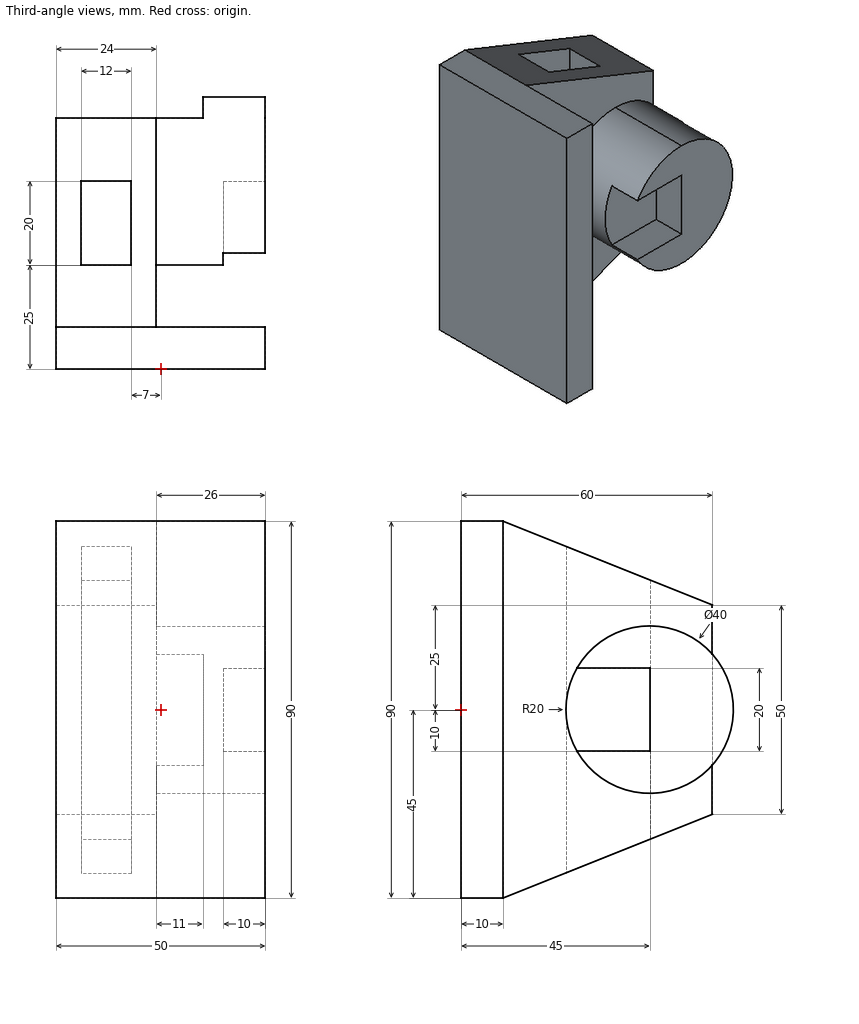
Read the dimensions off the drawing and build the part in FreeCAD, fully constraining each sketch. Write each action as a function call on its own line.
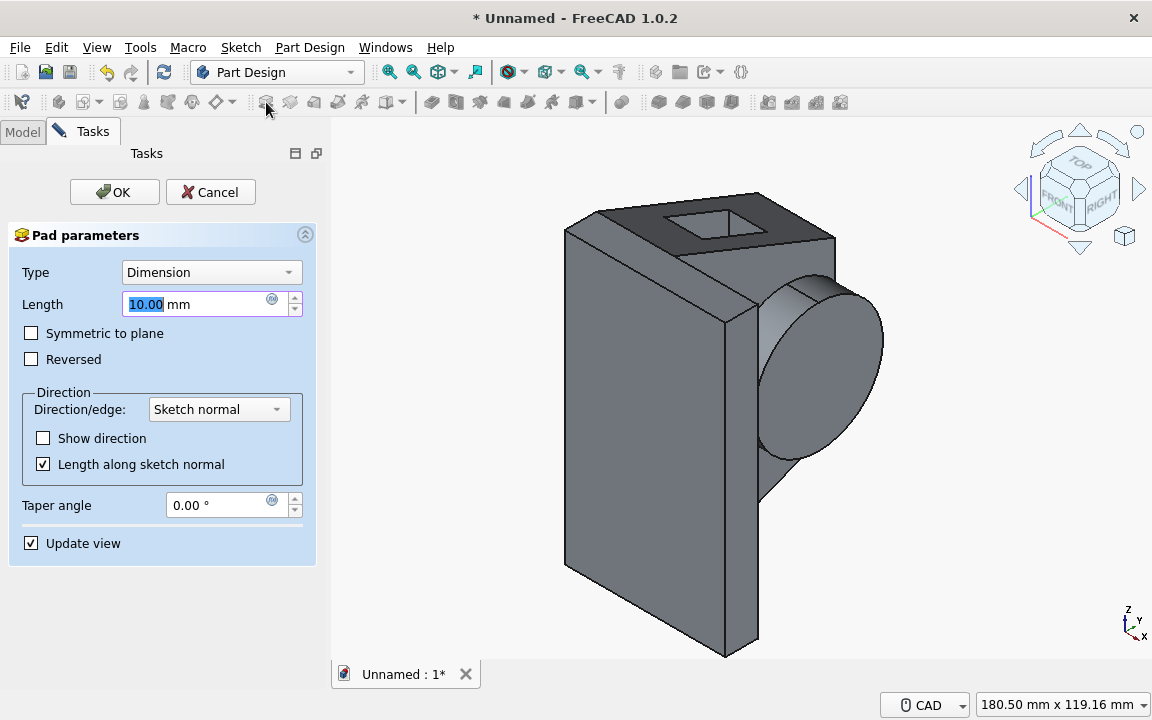
text(26)
key(Tab)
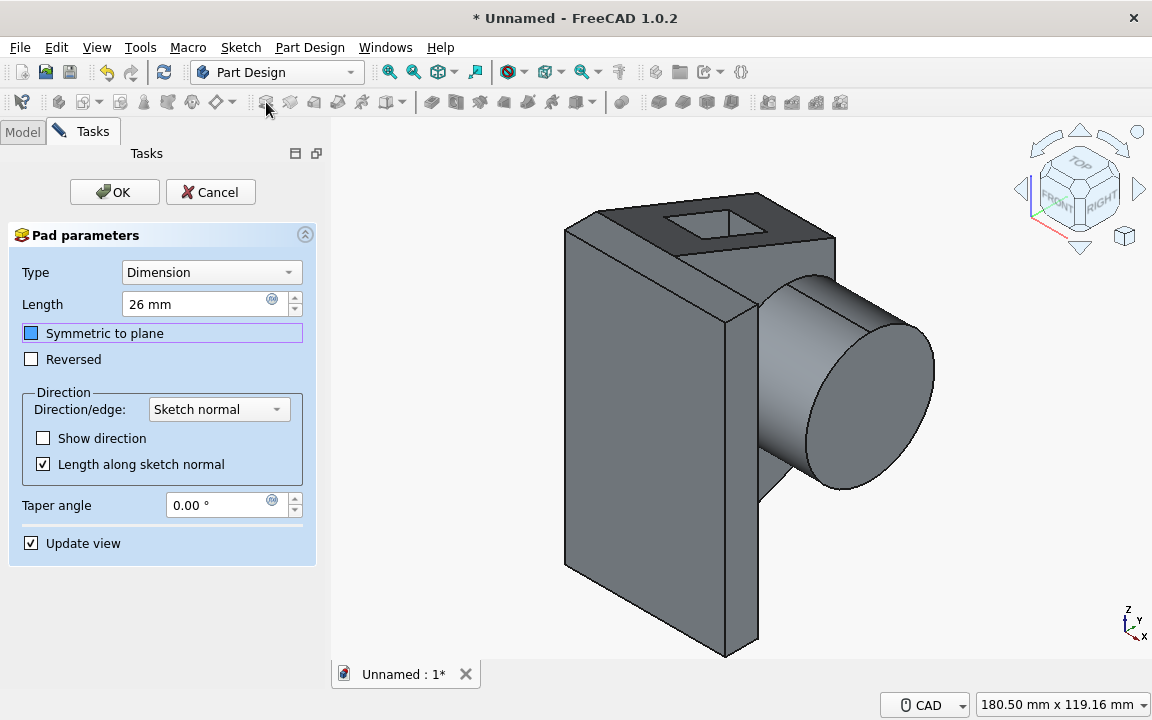
click(115, 192)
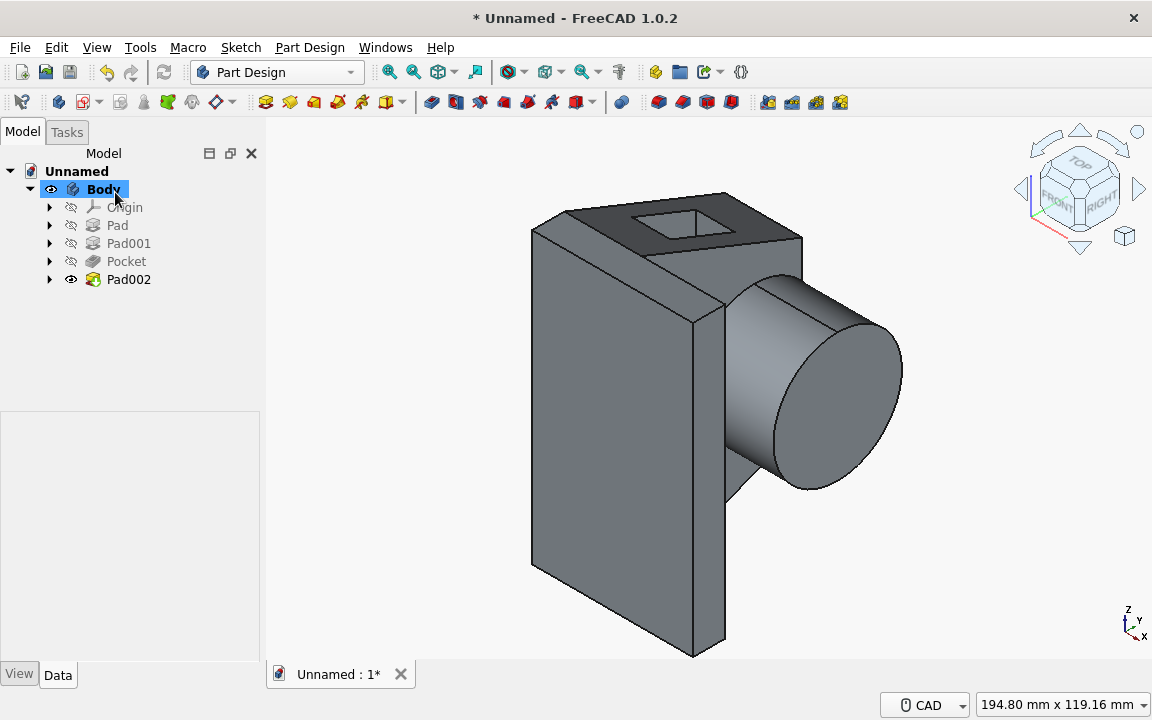
click(390, 72)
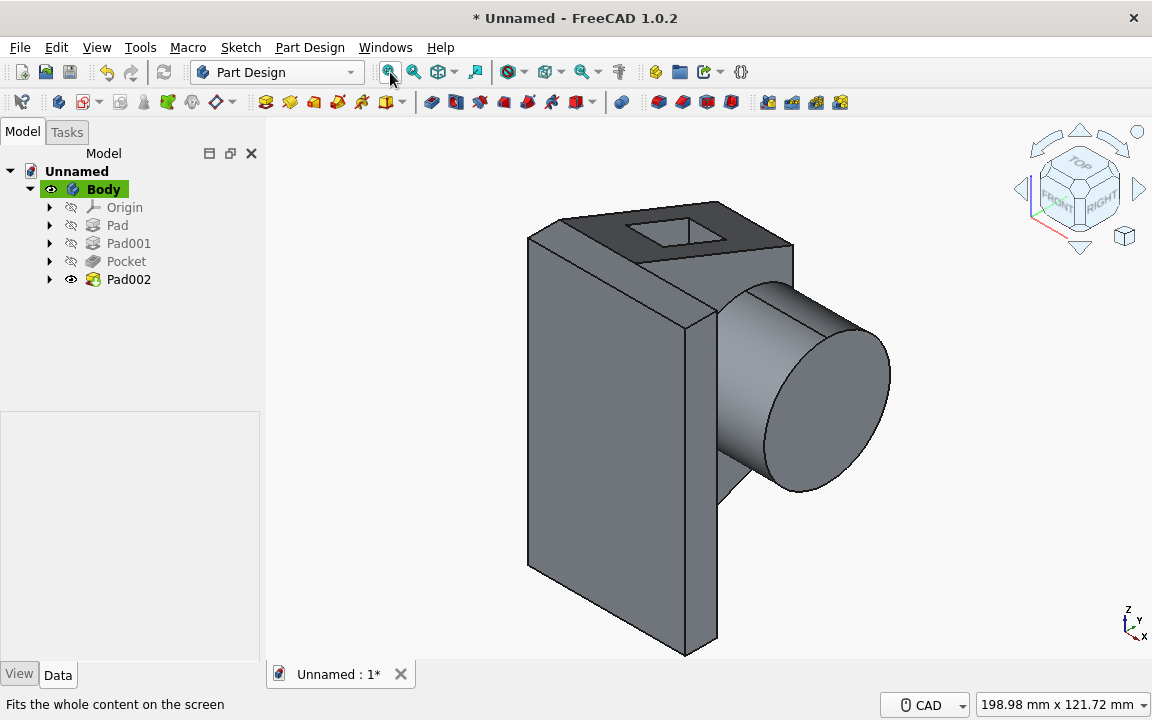
click(50, 207)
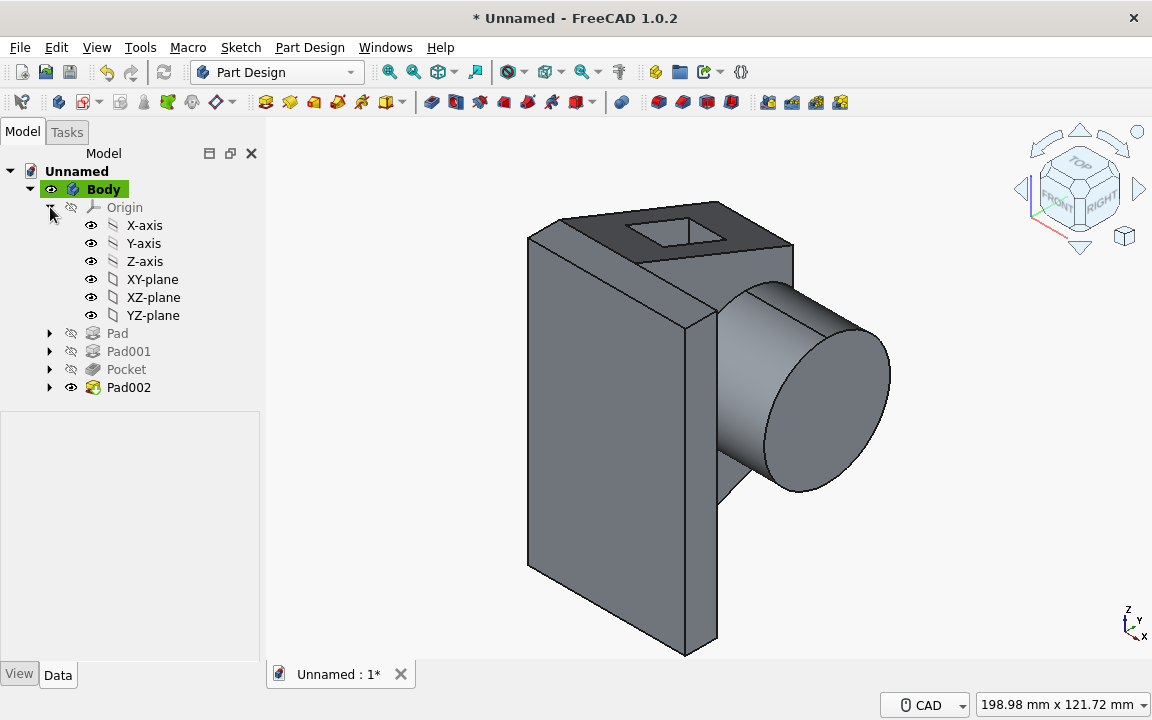
click(136, 315)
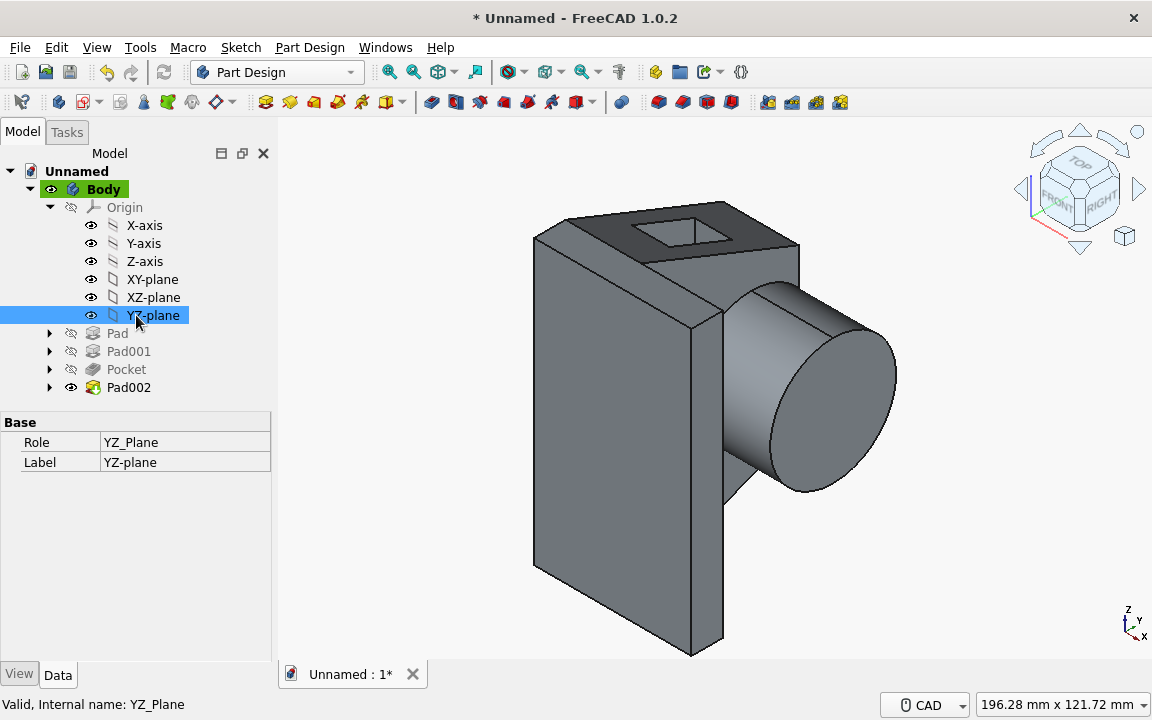
click(216, 102)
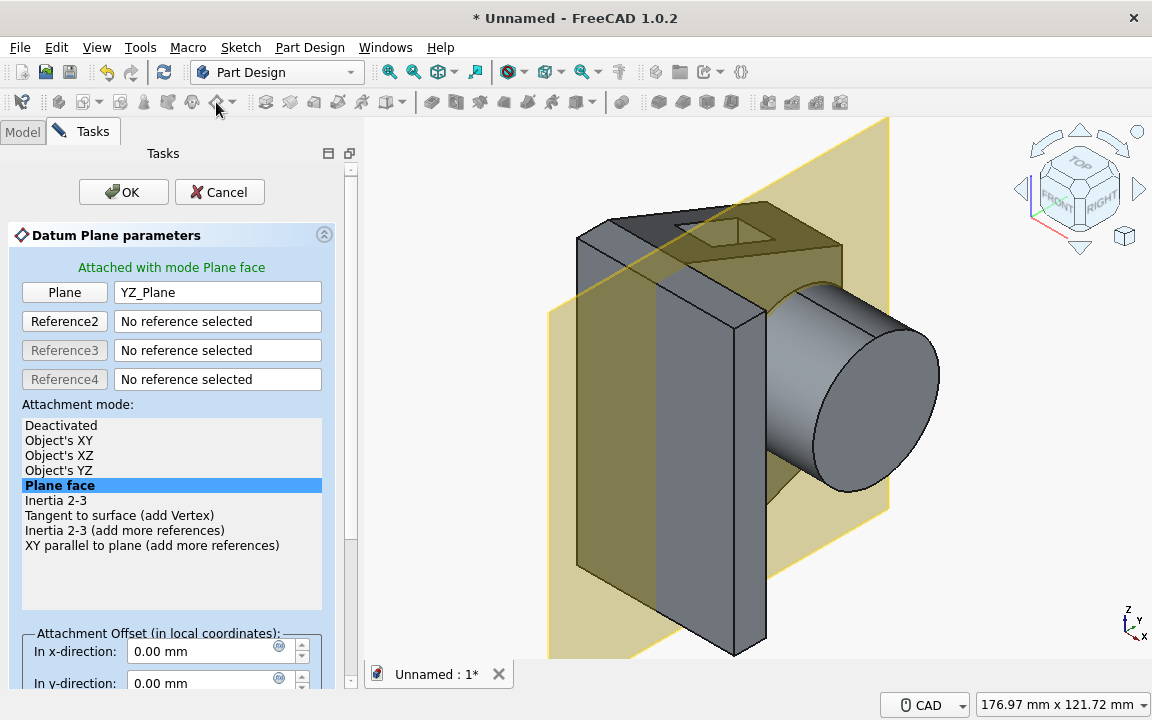
scroll(351, 426, down, 2)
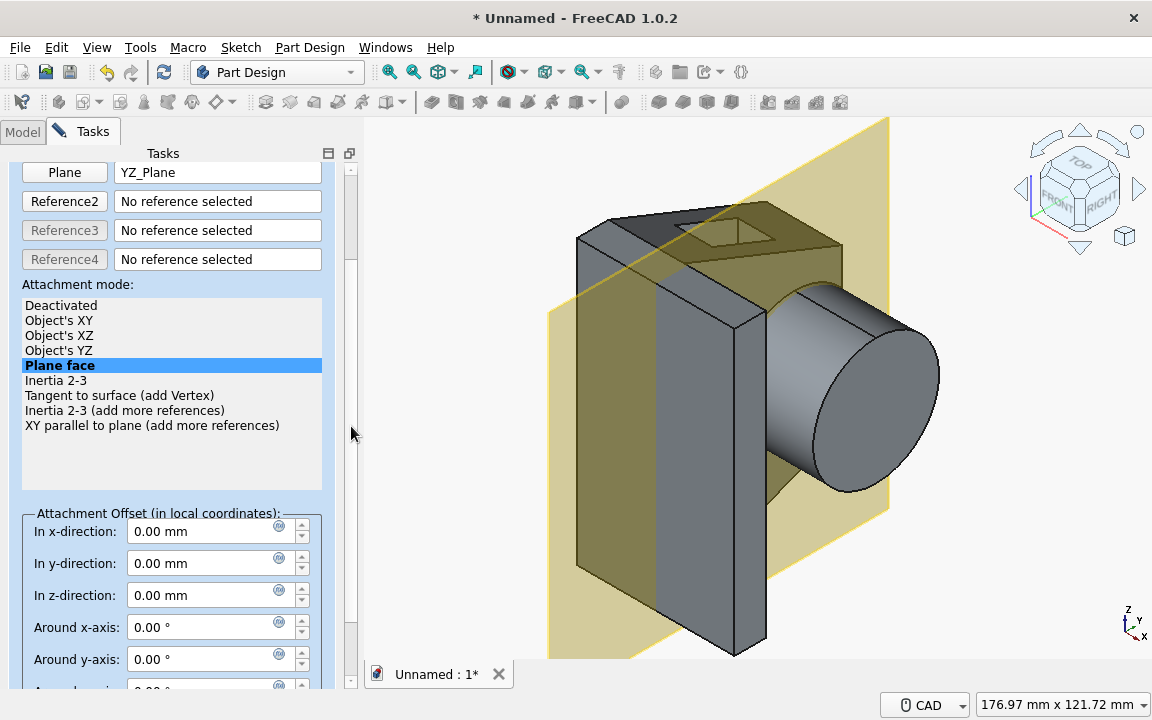
triple_click(210, 595)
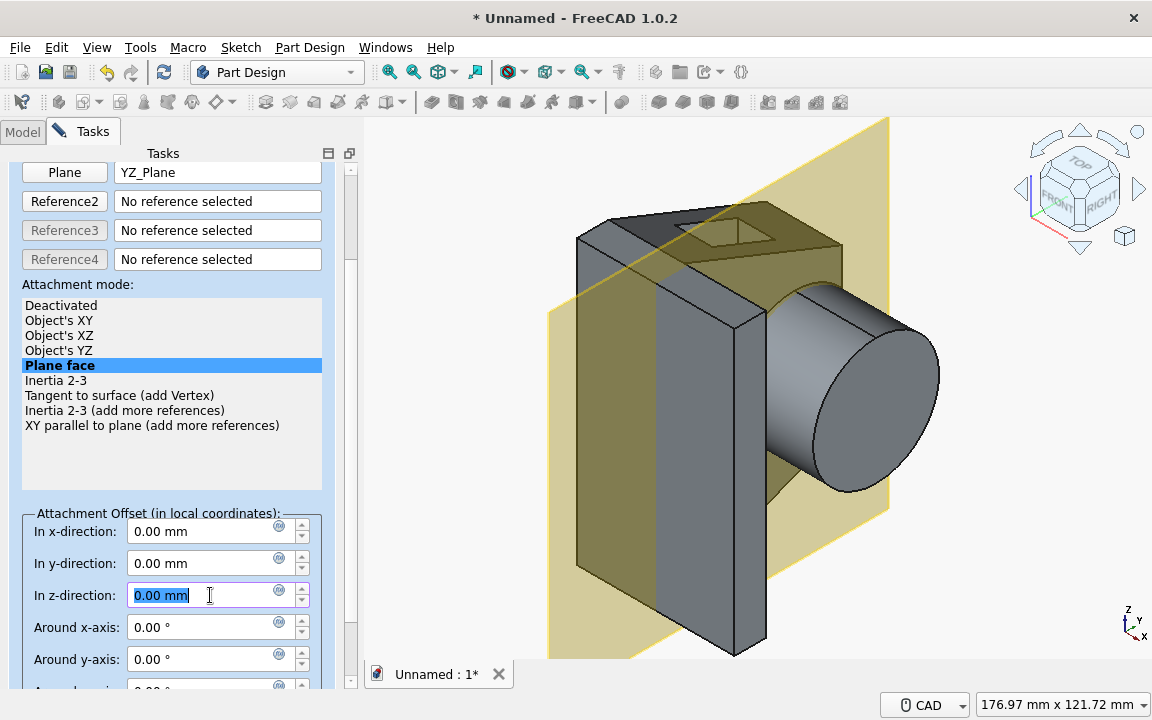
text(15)
key(Tab)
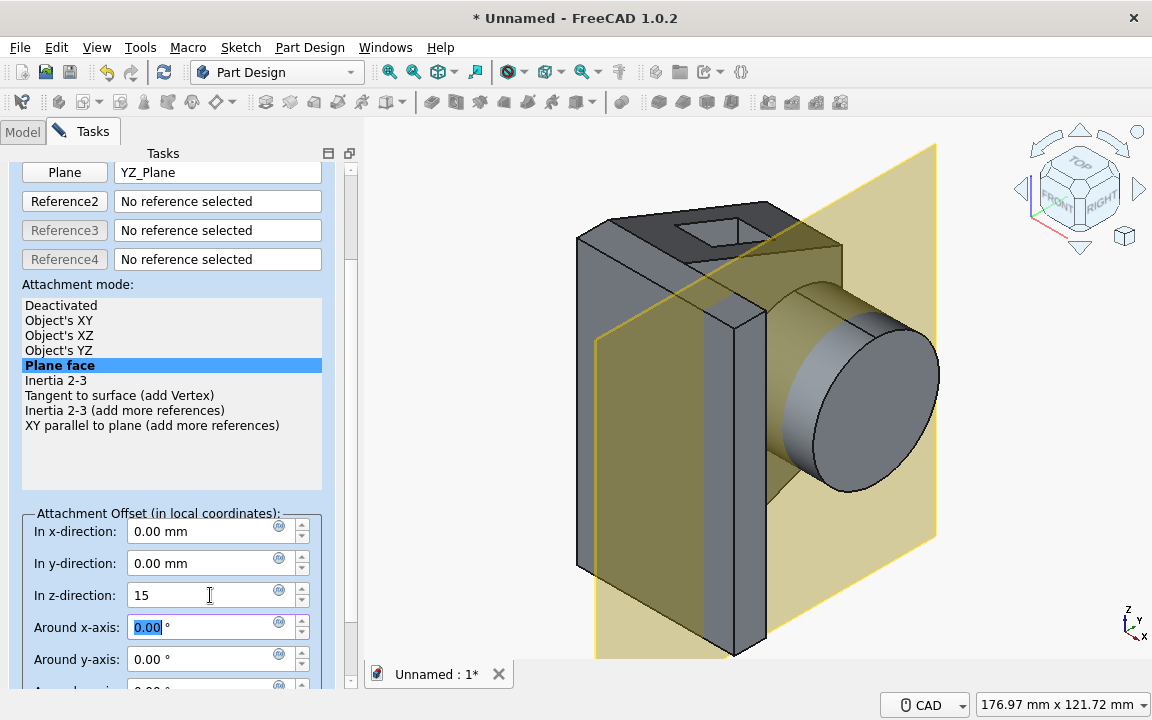
scroll(351, 426, up, 3)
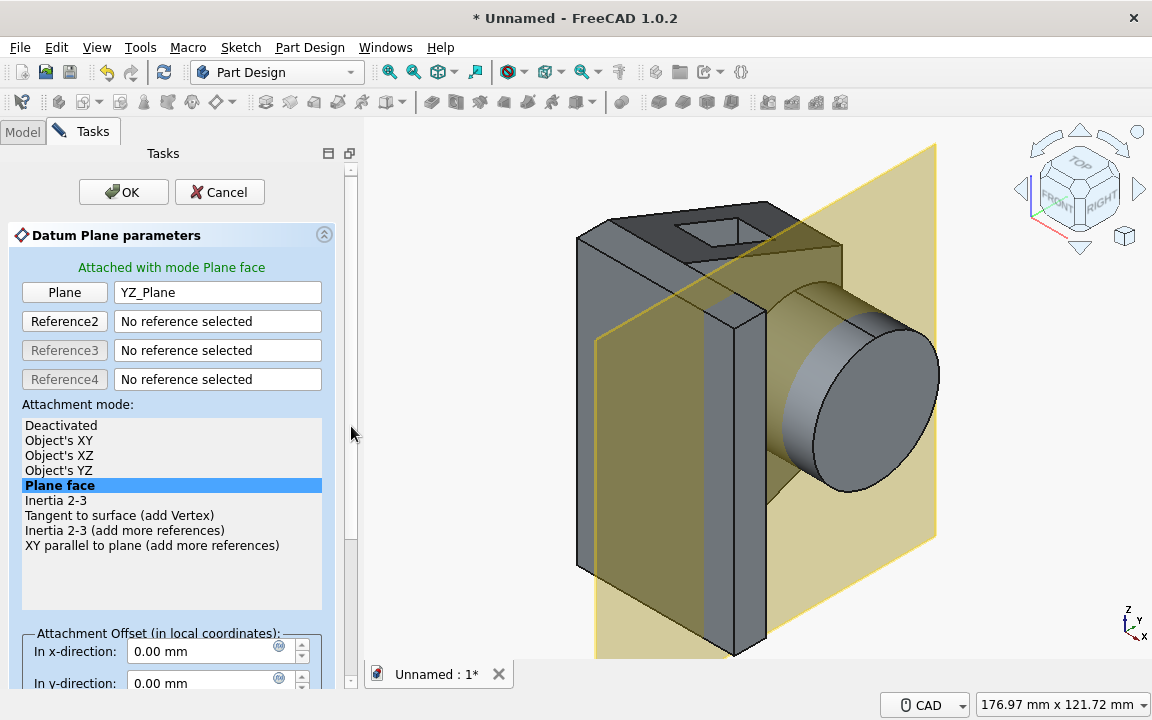
click(124, 192)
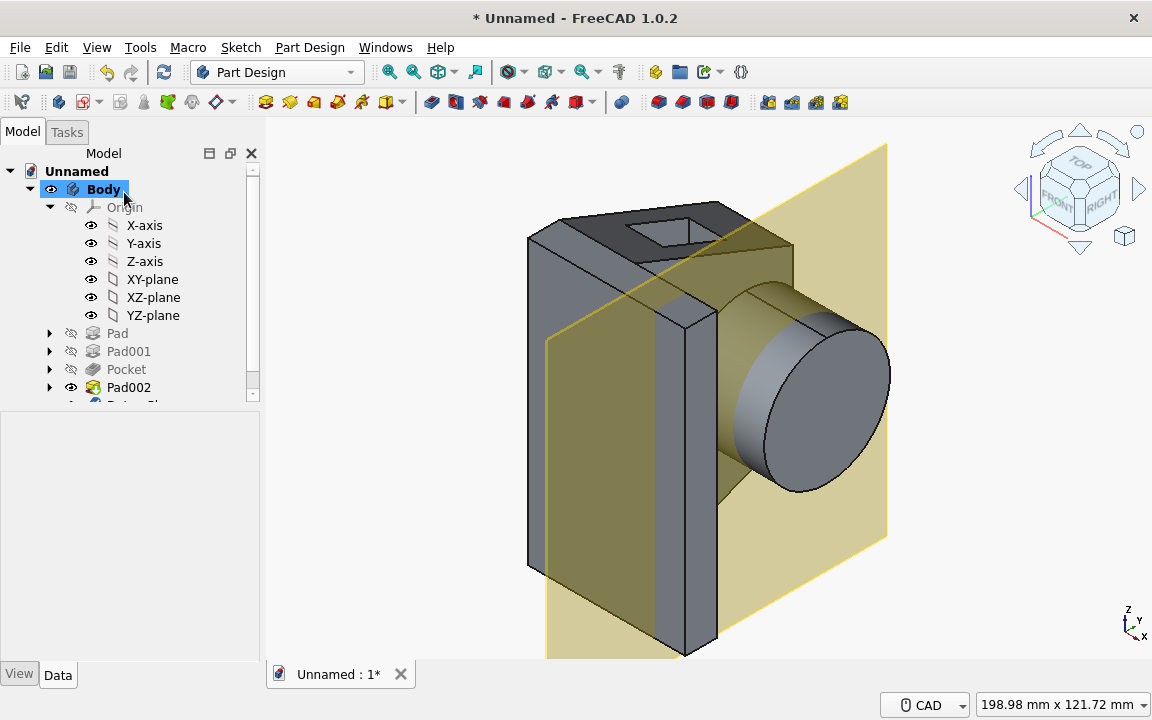
scroll(100, 275, down, 3)